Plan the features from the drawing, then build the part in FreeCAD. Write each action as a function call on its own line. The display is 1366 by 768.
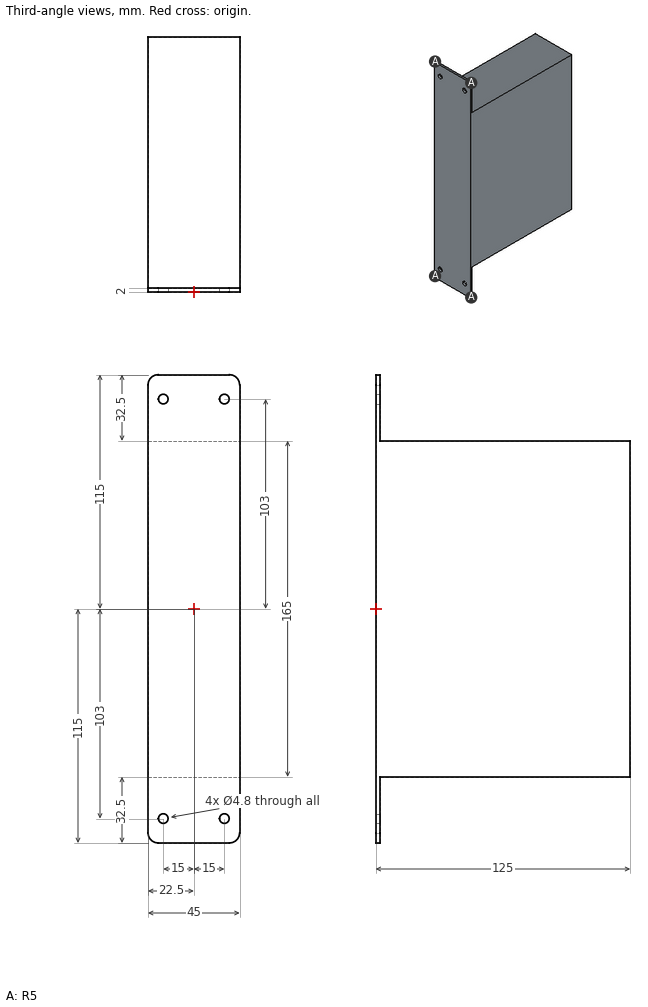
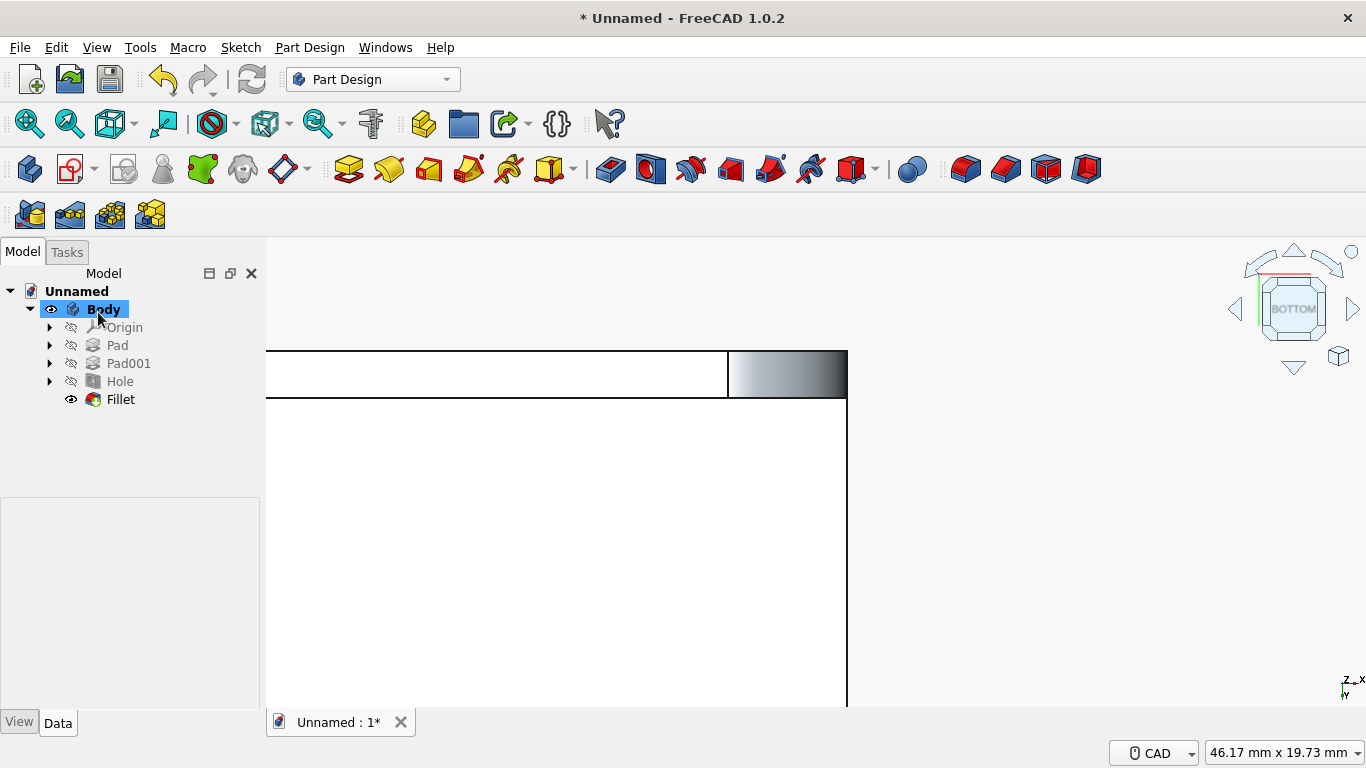
key(0)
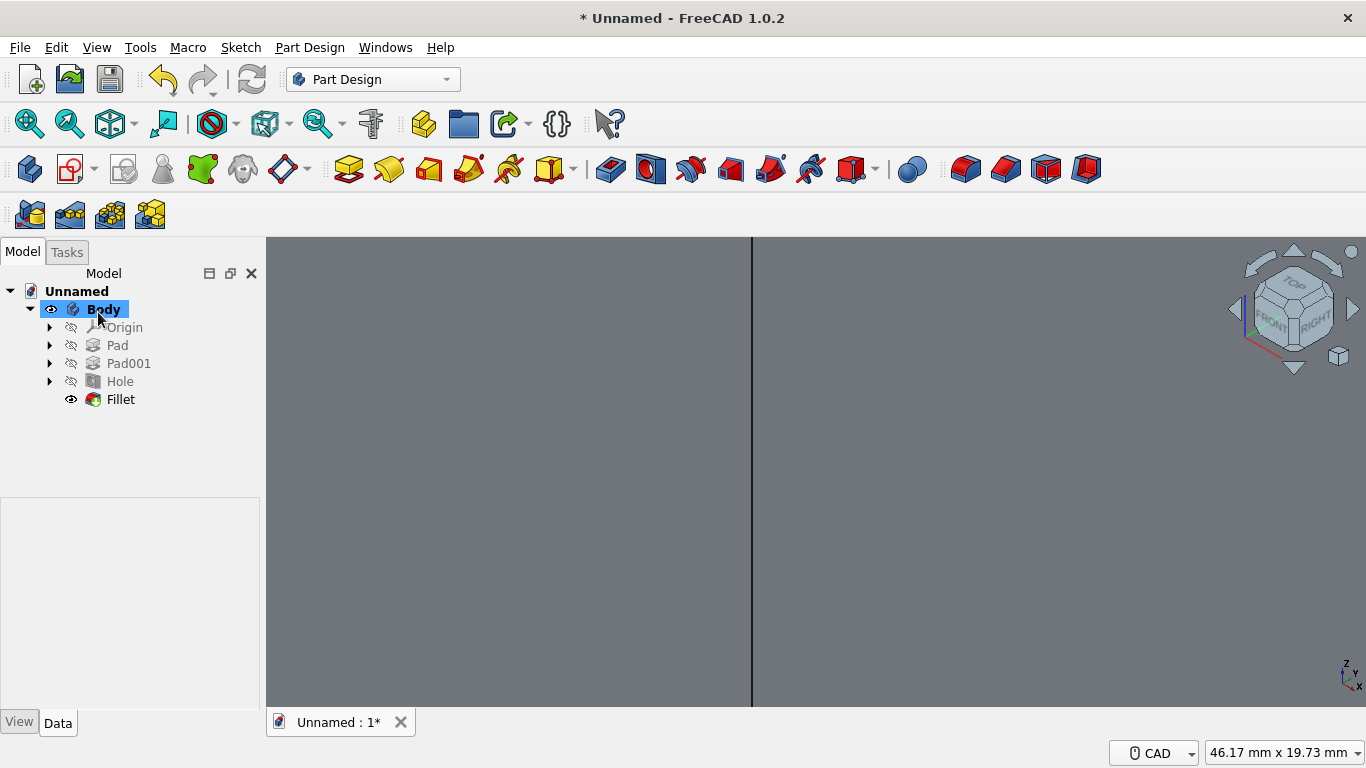
click(30, 124)